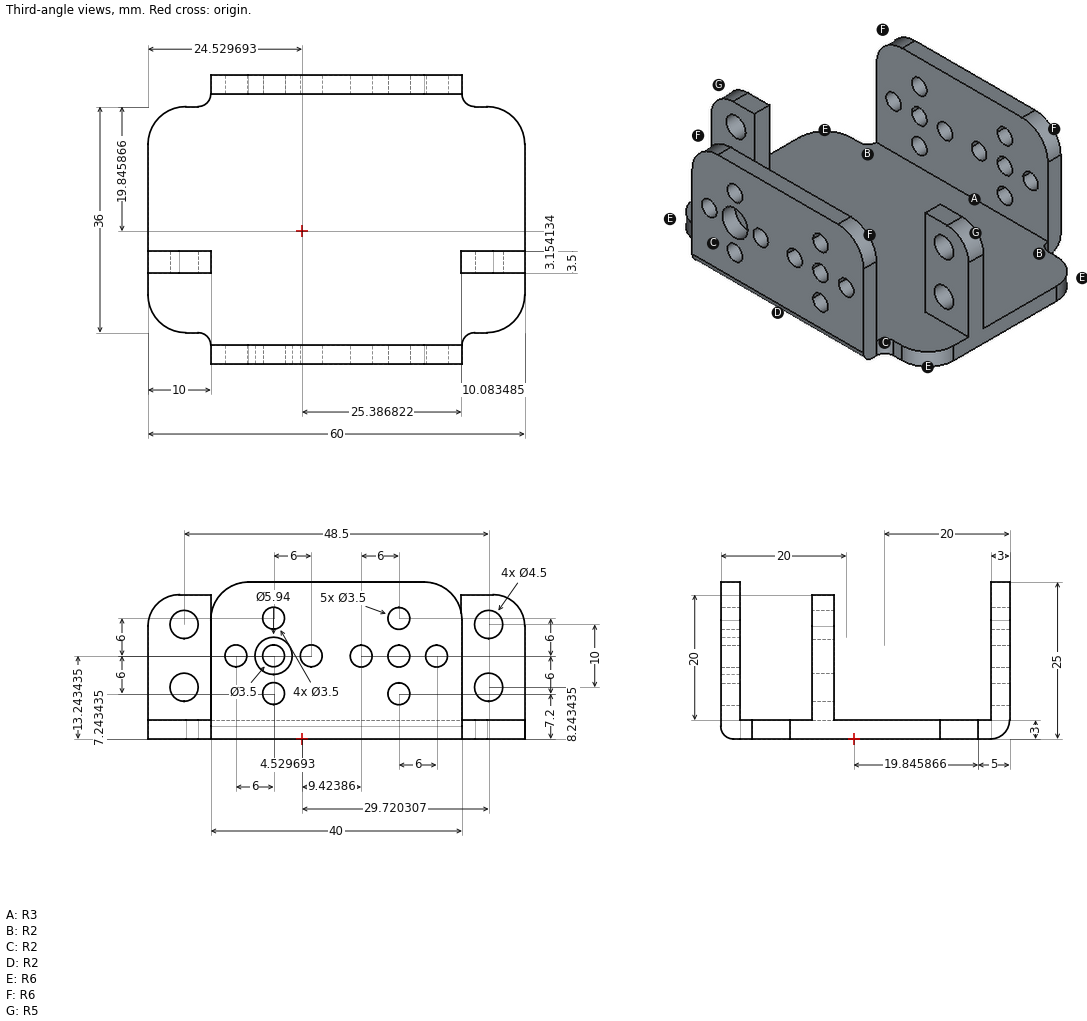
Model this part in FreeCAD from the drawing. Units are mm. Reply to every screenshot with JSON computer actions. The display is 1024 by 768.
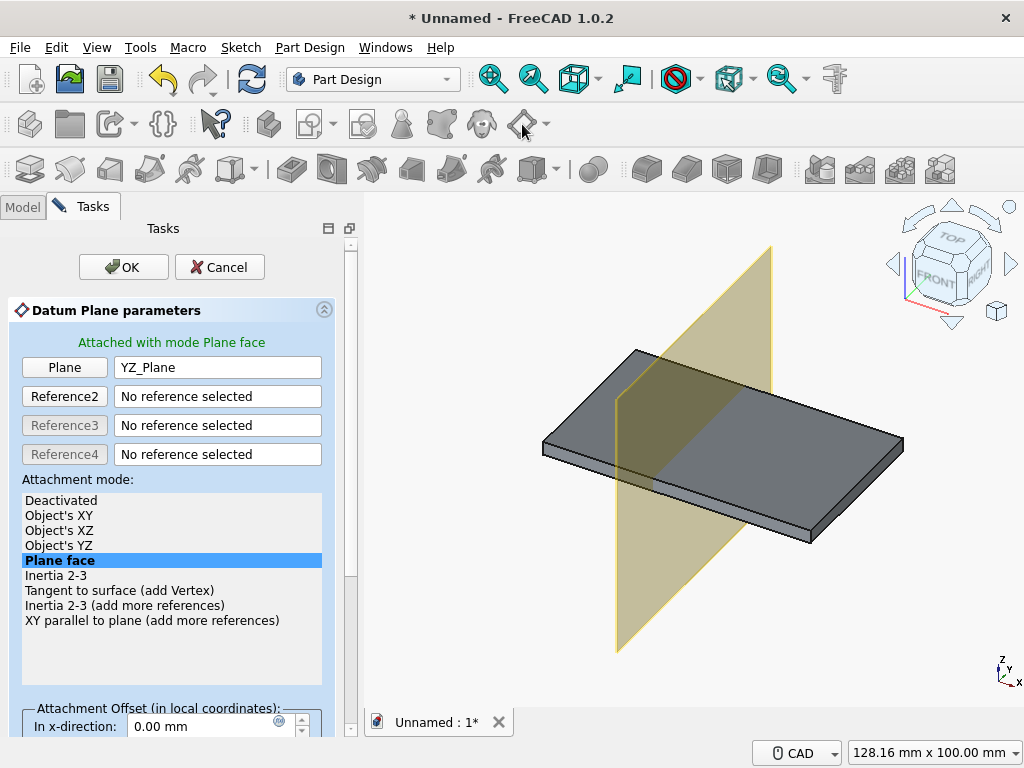
{"action": "scroll", "coordinate": [351, 487], "scroll_direction": "down", "scroll_amount": 3}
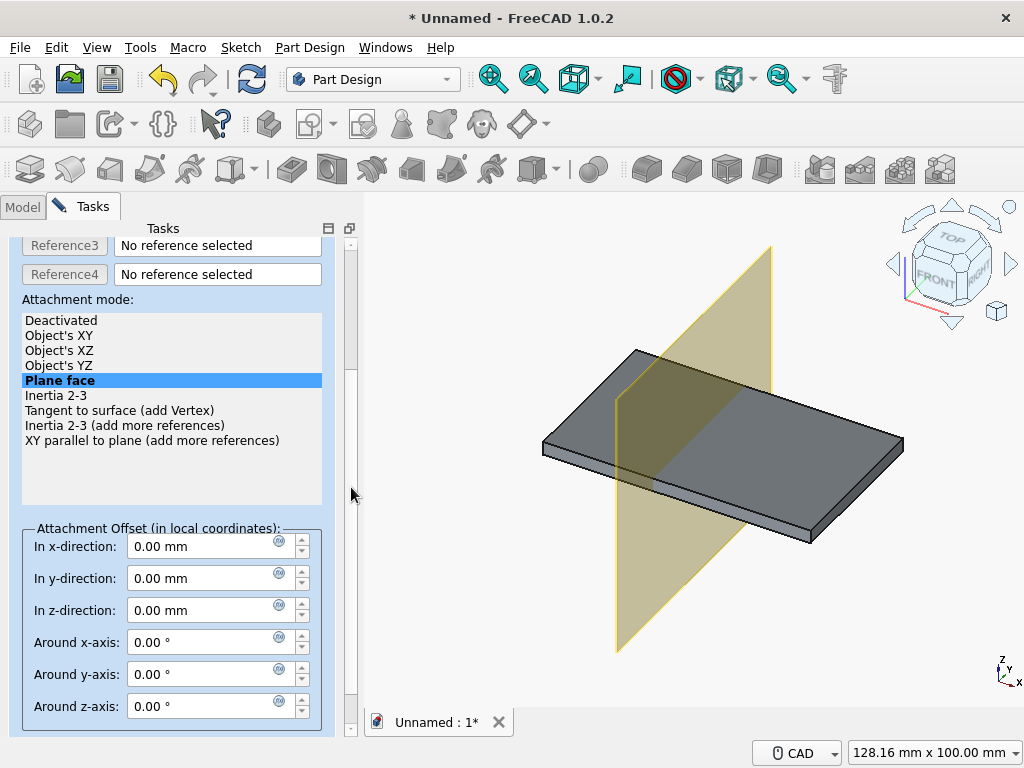
{"action": "triple_click", "coordinate": [210, 610]}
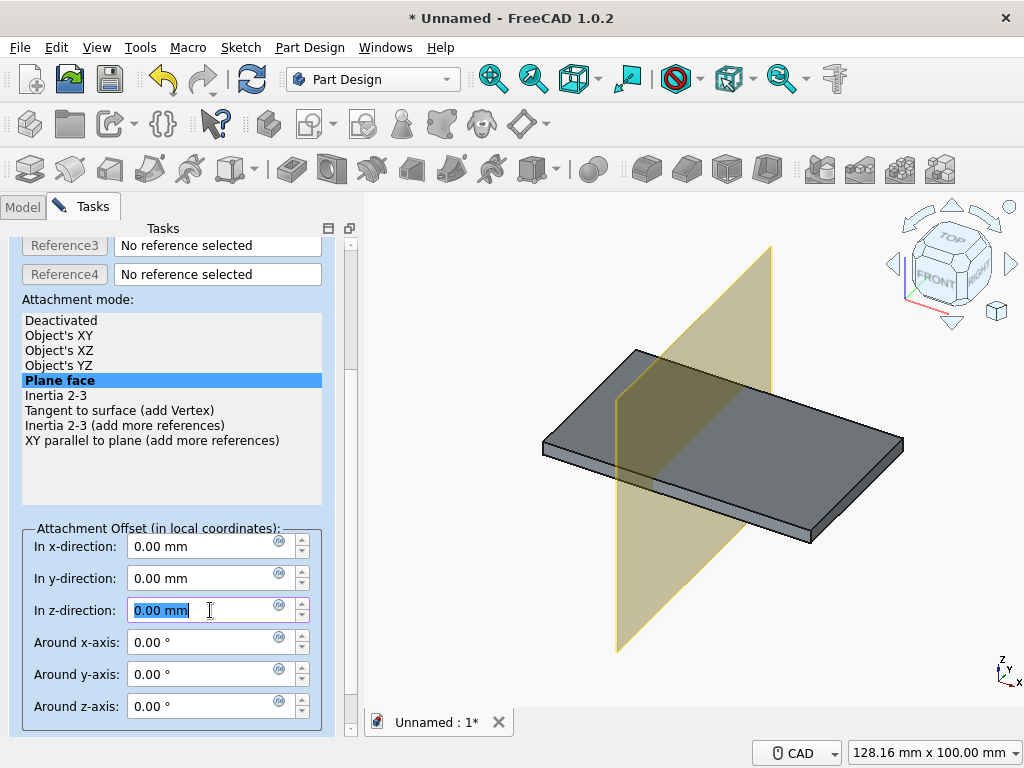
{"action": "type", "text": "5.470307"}
{"action": "key", "text": "Tab"}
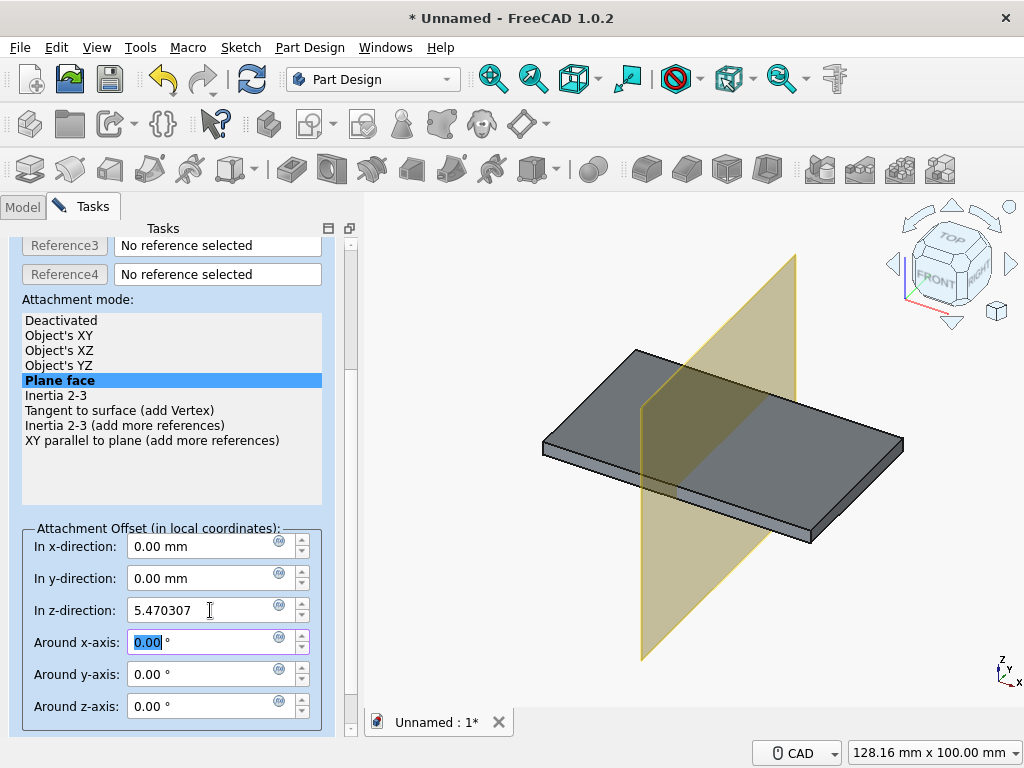
{"action": "scroll", "coordinate": [351, 487], "scroll_direction": "up", "scroll_amount": 4}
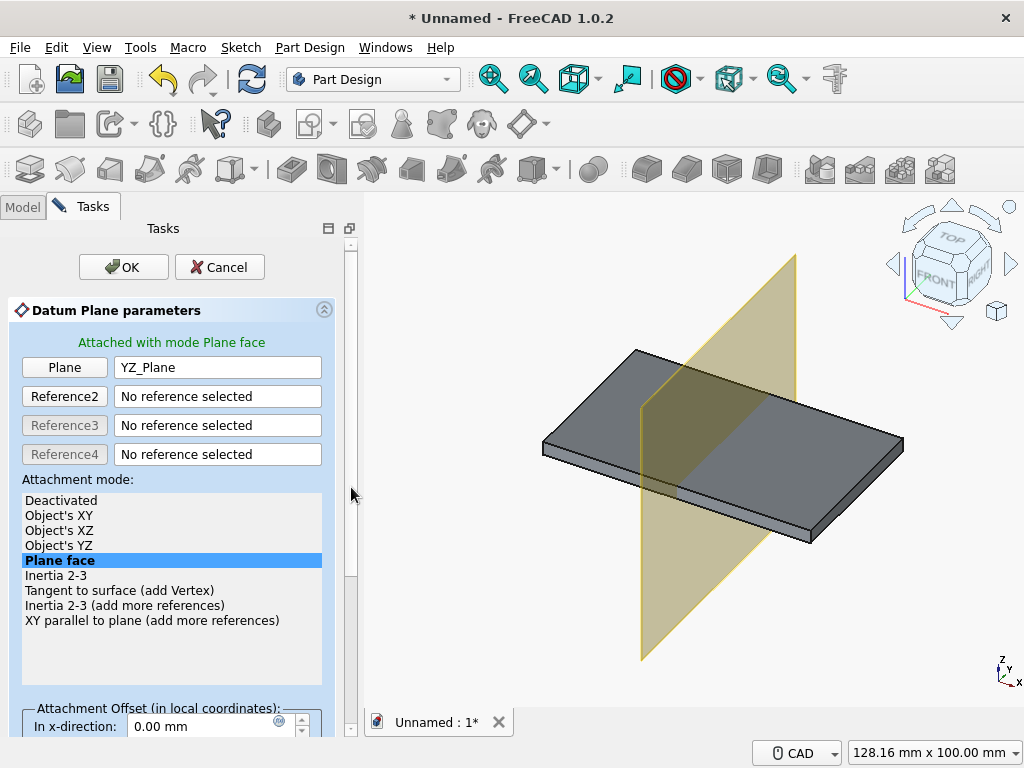
{"action": "left_click", "coordinate": [124, 267]}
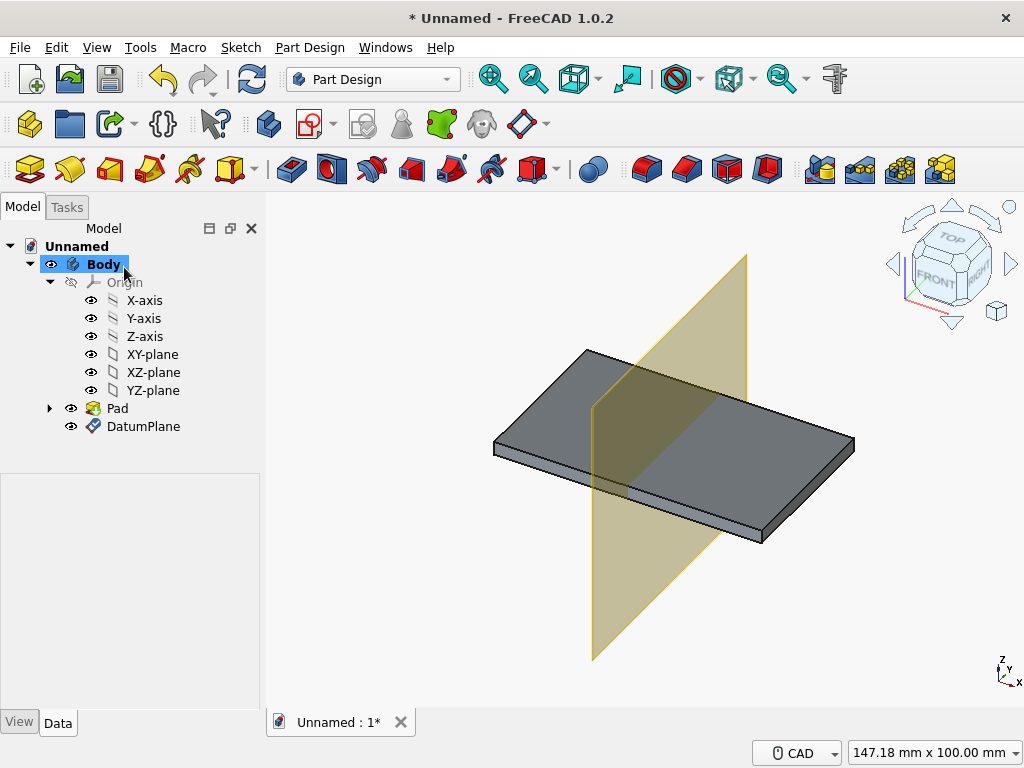
{"action": "left_click", "coordinate": [116, 426]}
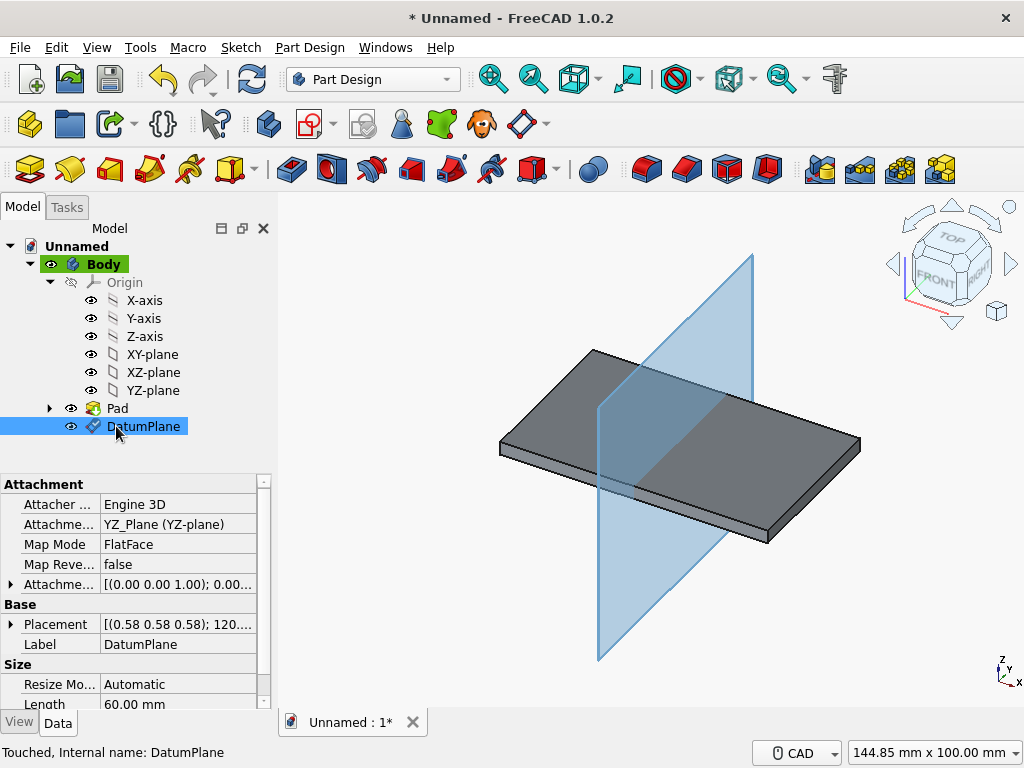
{"action": "left_click", "coordinate": [310, 124]}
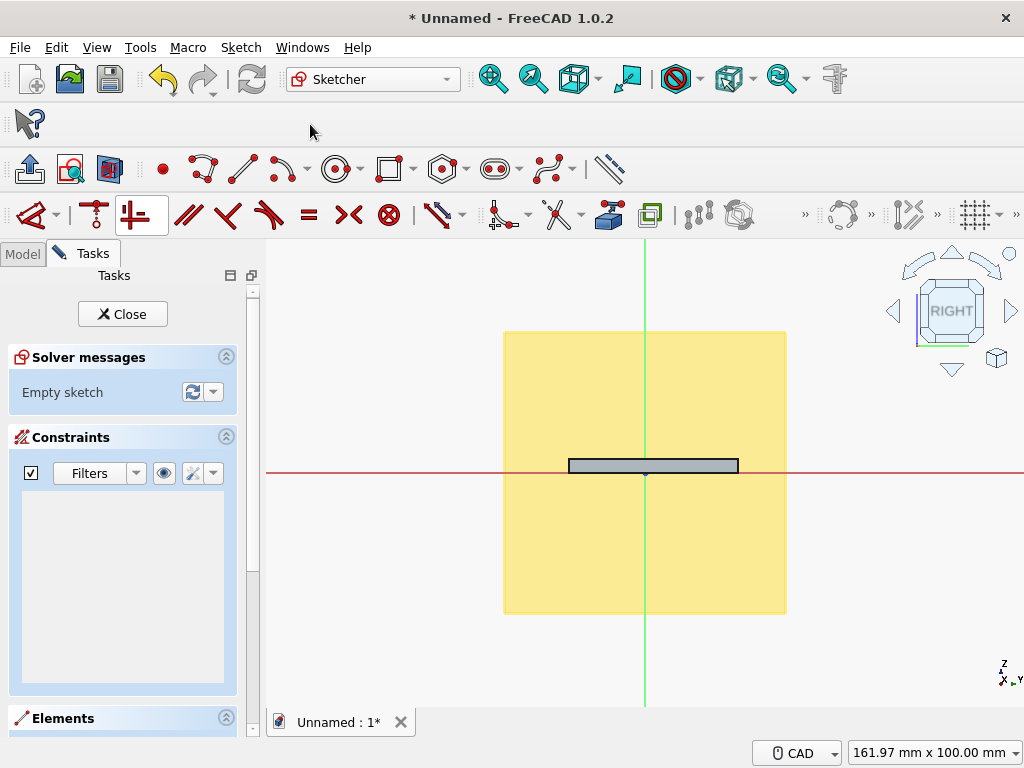
{"action": "left_click", "coordinate": [110, 170]}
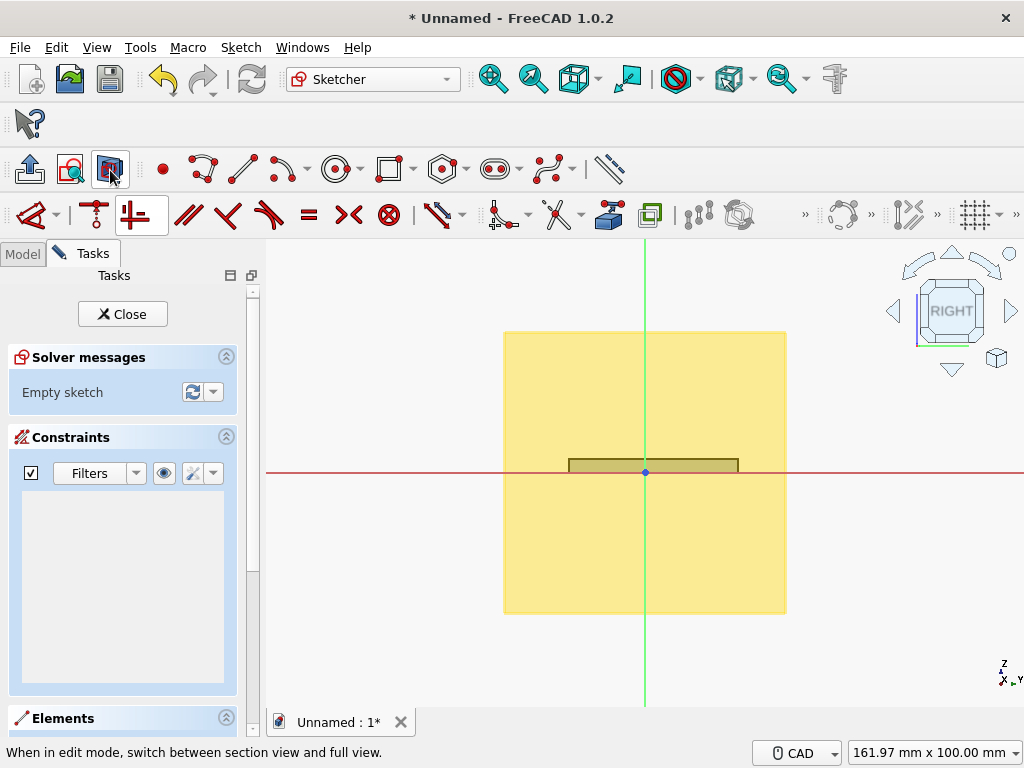
{"action": "scroll", "coordinate": [777, 380], "scroll_direction": "up", "scroll_amount": 5}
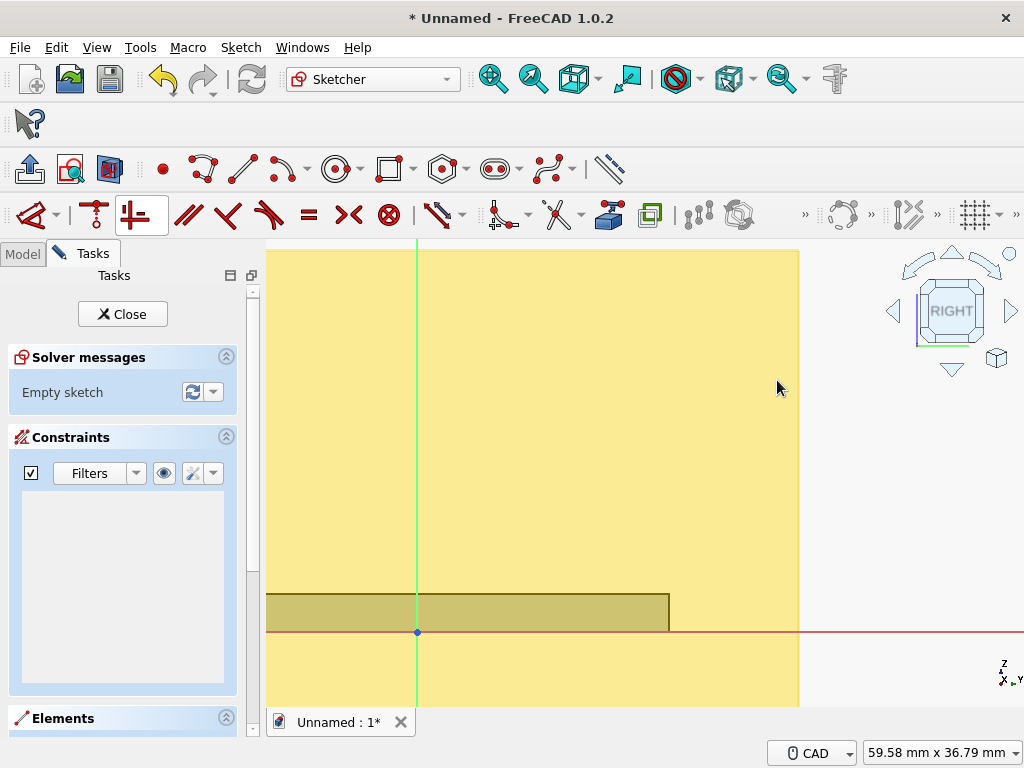
{"action": "left_click", "coordinate": [204, 170]}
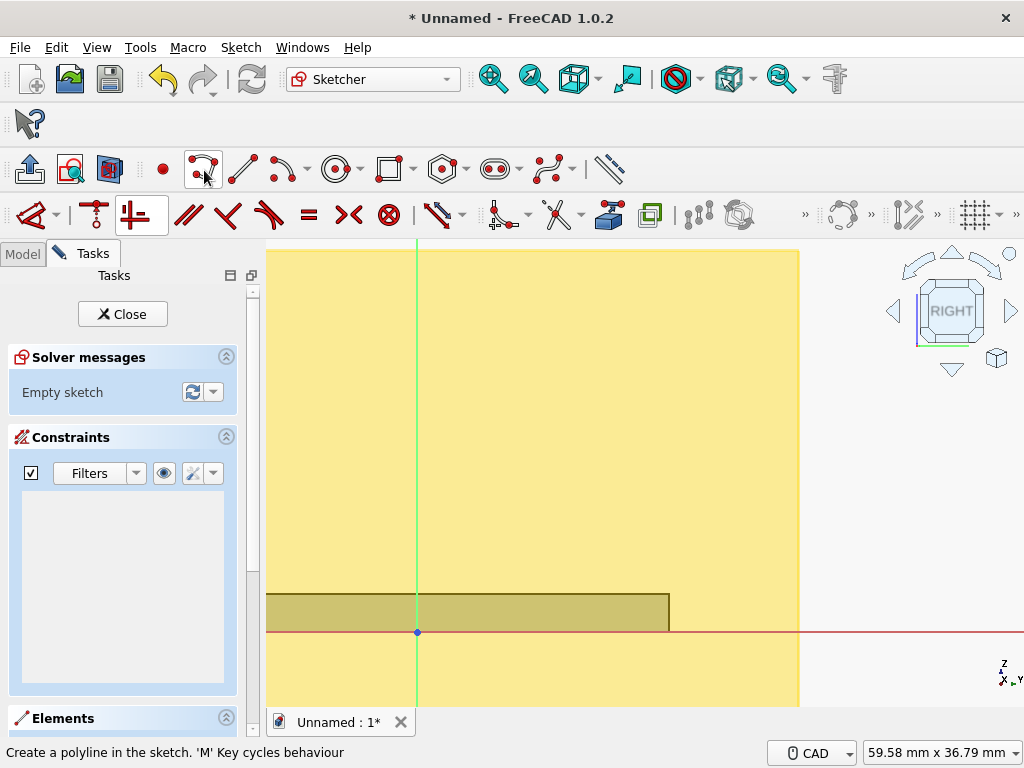
{"action": "left_click", "coordinate": [669, 632]}
{"action": "left_click", "coordinate": [733, 623]}
{"action": "left_click", "coordinate": [733, 314]}
{"action": "left_click", "coordinate": [695, 314]}
{"action": "left_click", "coordinate": [695, 594]}
{"action": "left_click", "coordinate": [669, 594]}
{"action": "left_click", "coordinate": [669, 632]}
{"action": "key", "text": "Escape"}
{"action": "key", "text": "Escape"}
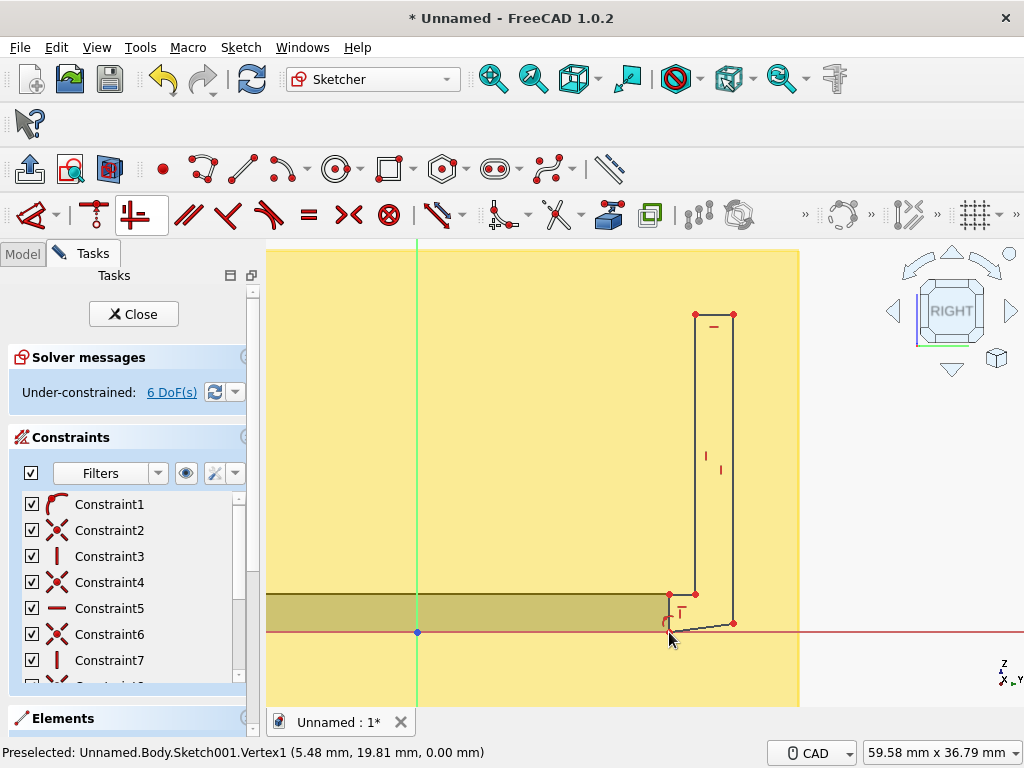
{"action": "left_click", "coordinate": [688, 630]}